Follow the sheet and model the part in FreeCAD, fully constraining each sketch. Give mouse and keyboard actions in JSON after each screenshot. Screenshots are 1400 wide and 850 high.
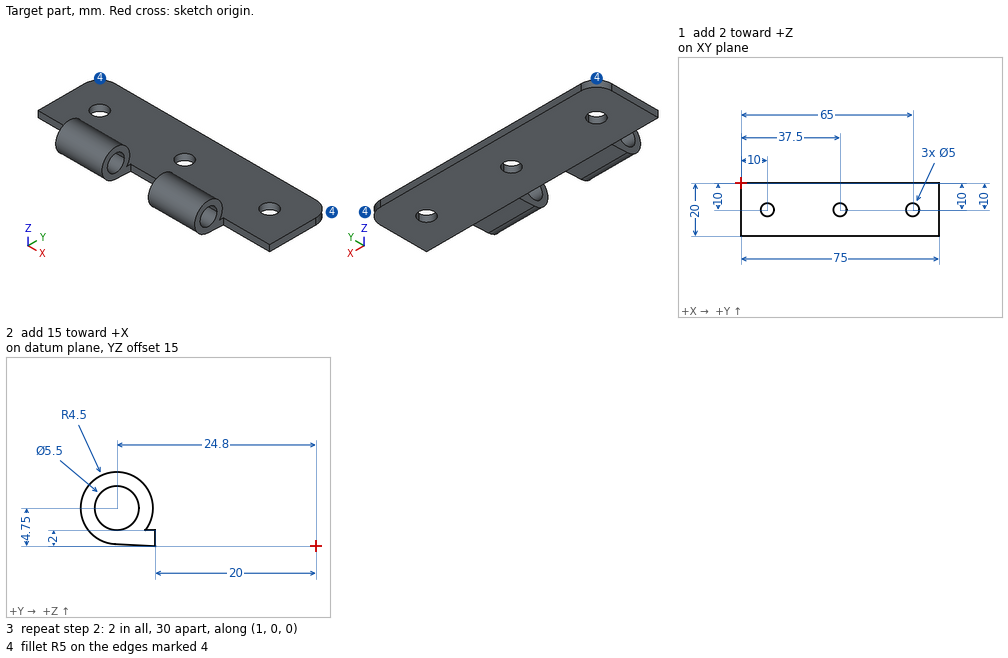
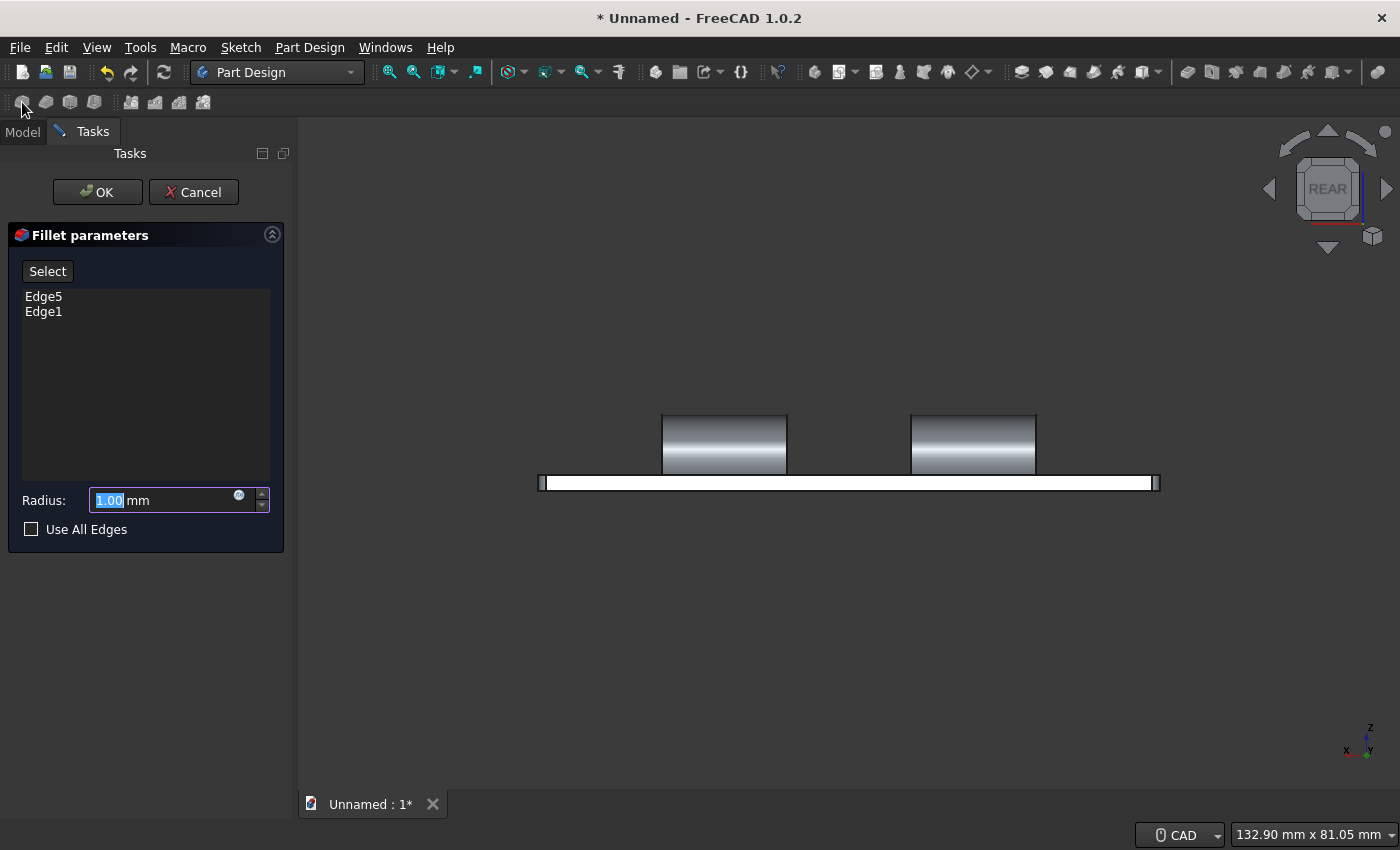
{"action": "type", "text": "5"}
{"action": "key", "text": "Tab"}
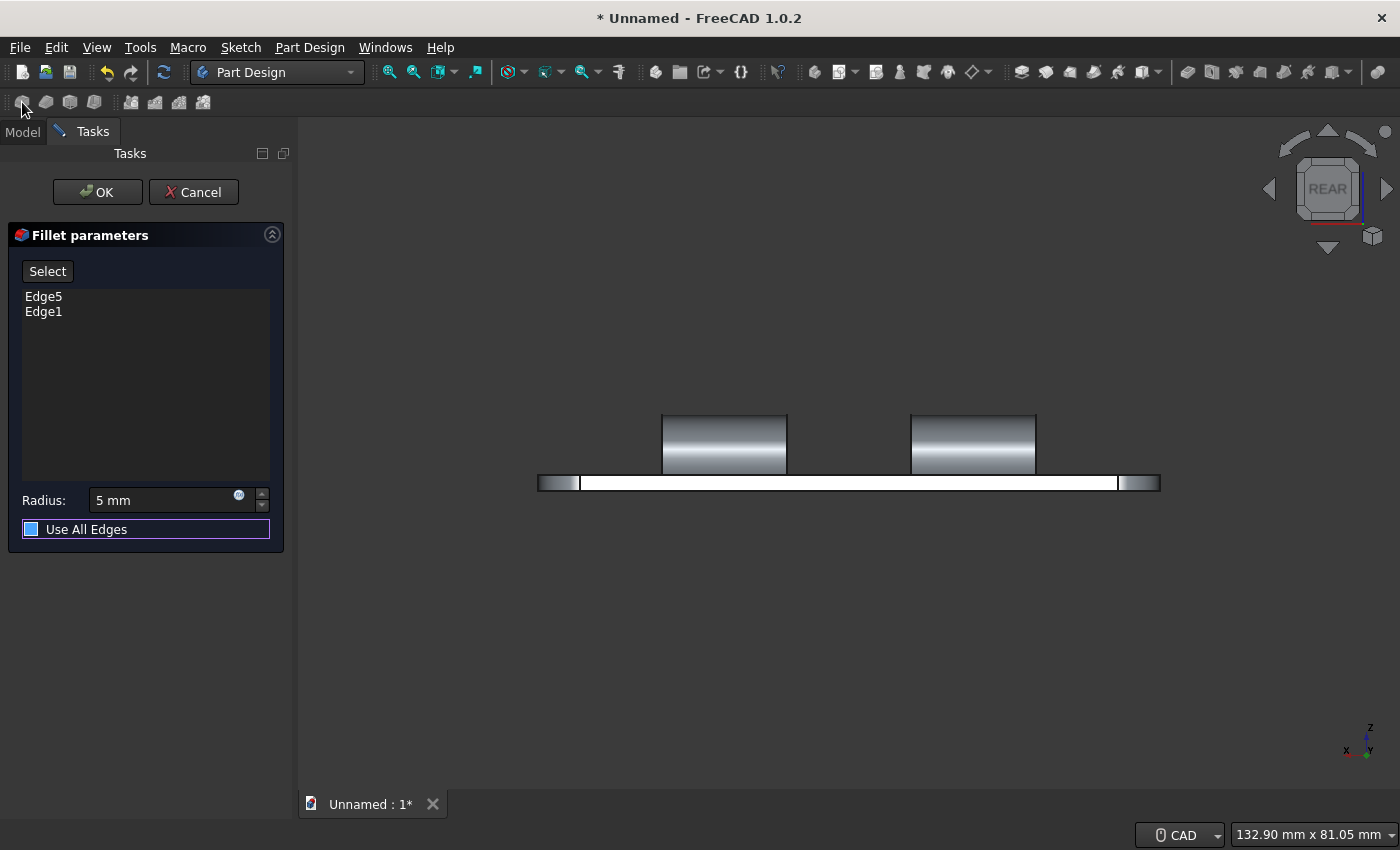
{"action": "left_click", "coordinate": [98, 192]}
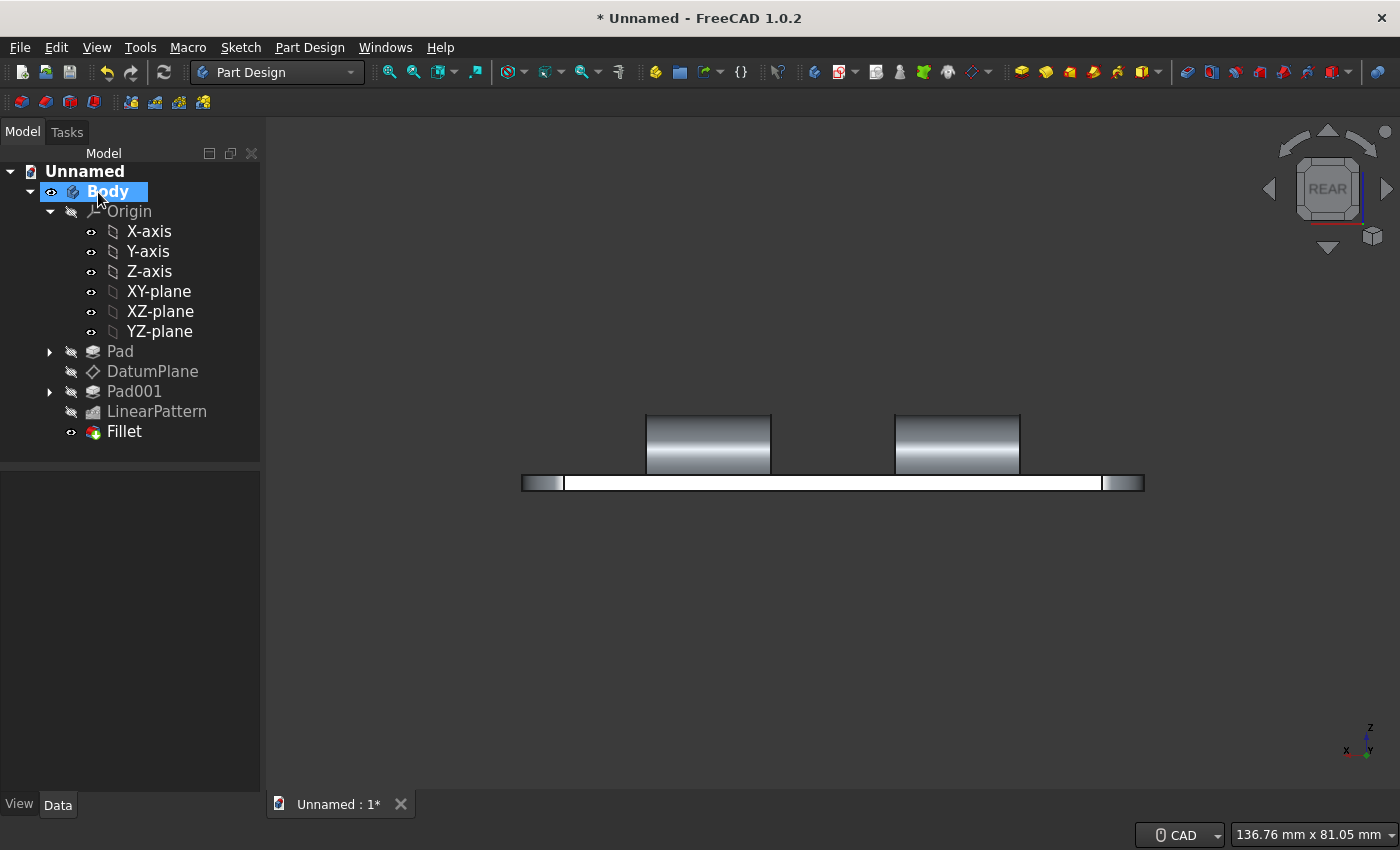
{"action": "key", "text": "0"}